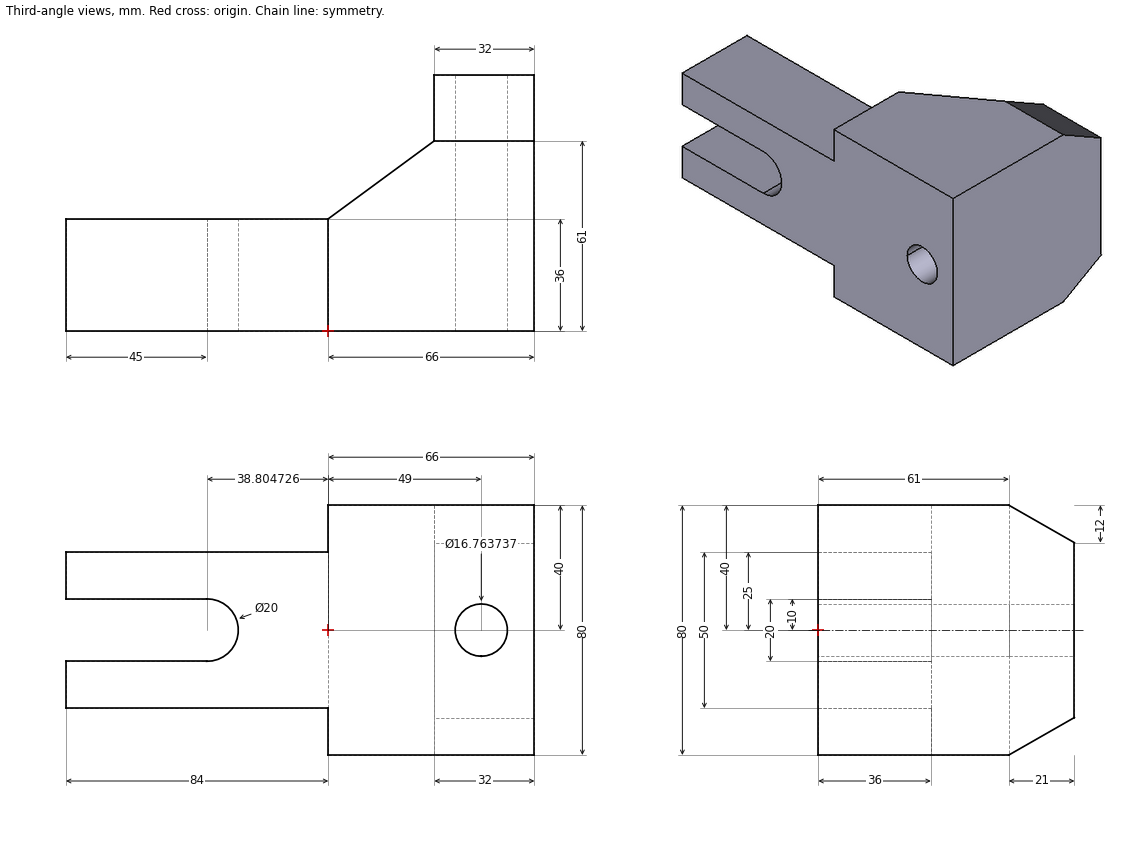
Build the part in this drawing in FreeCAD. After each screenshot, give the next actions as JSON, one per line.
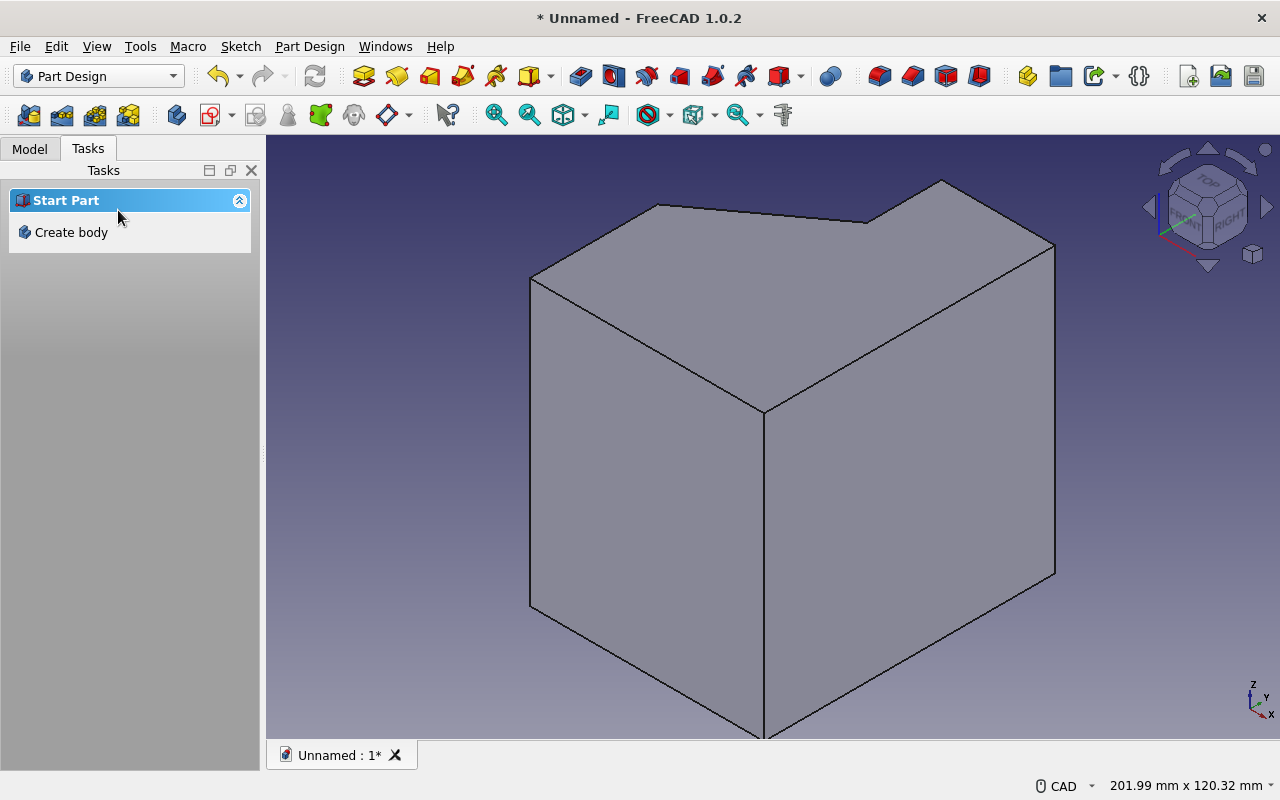
{"action": "left_click", "coordinate": [497, 116]}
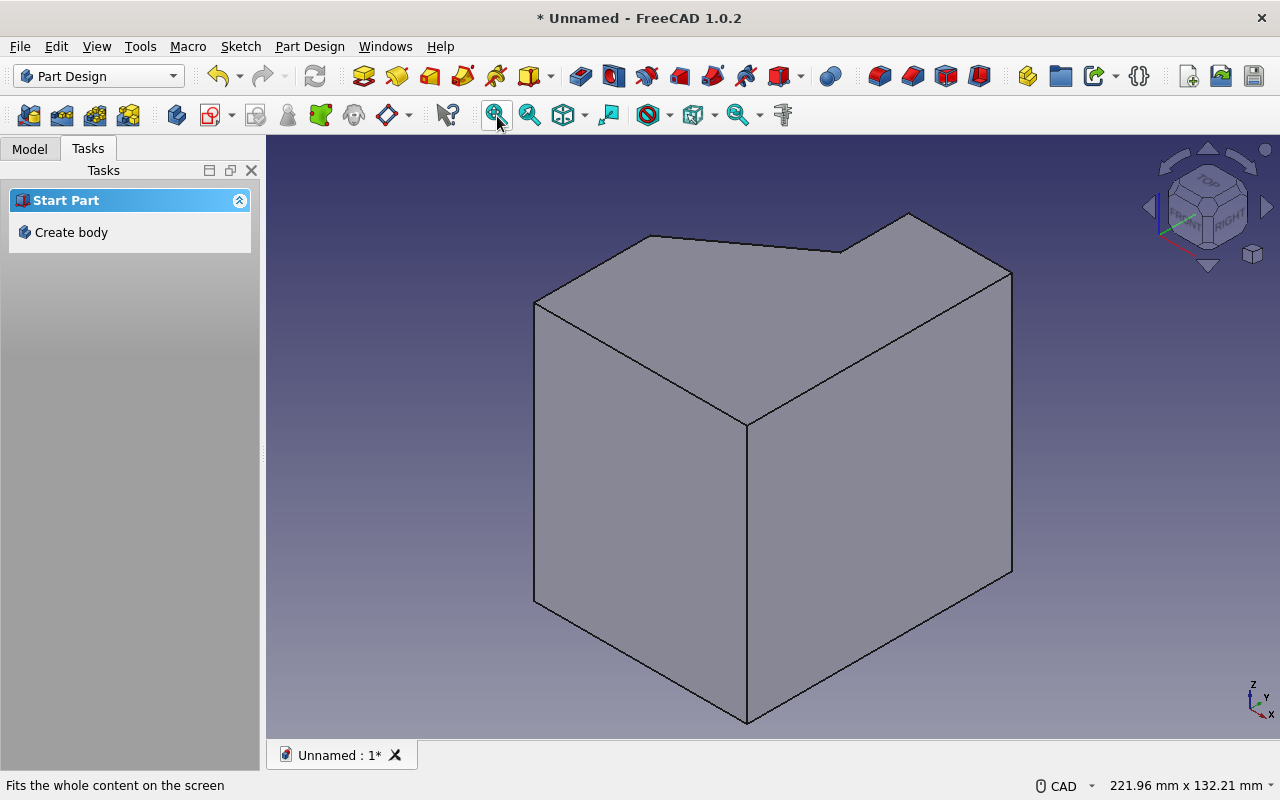
{"action": "left_click", "coordinate": [880, 498]}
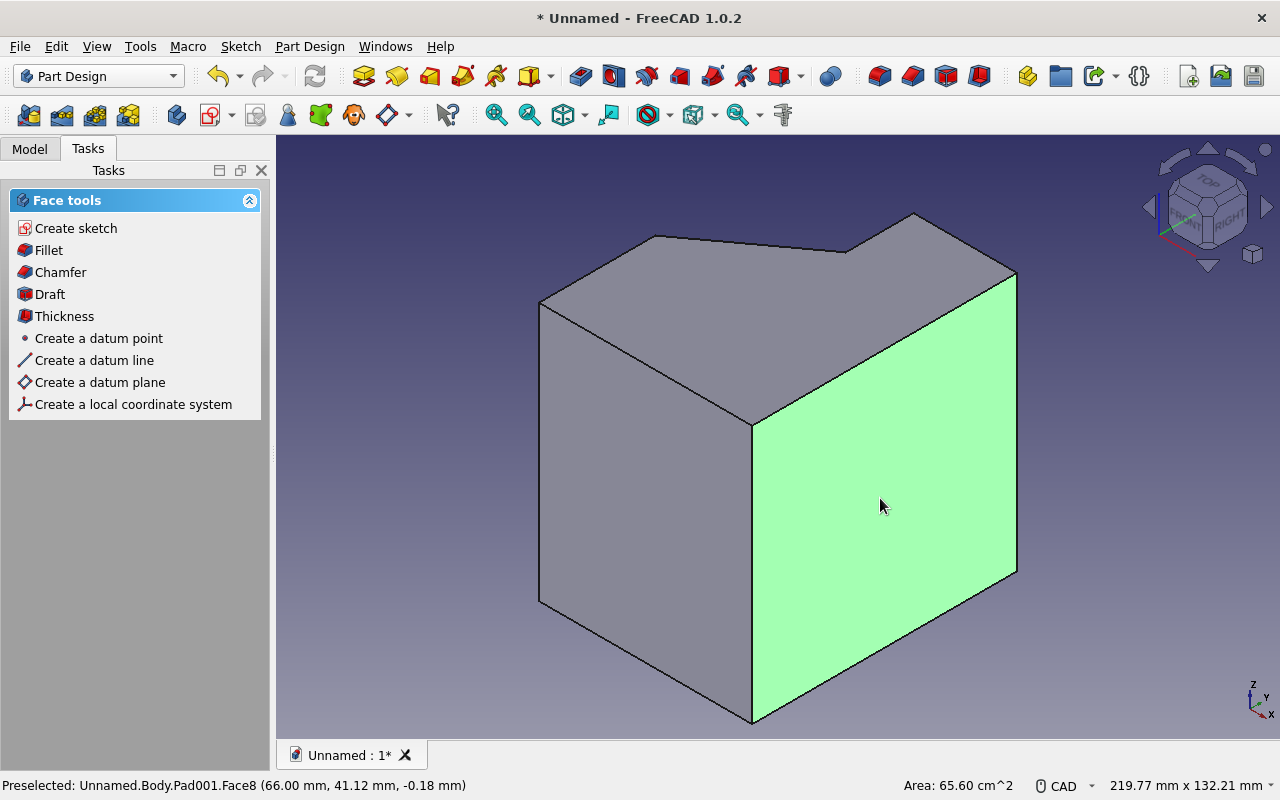
{"action": "left_click", "coordinate": [210, 116]}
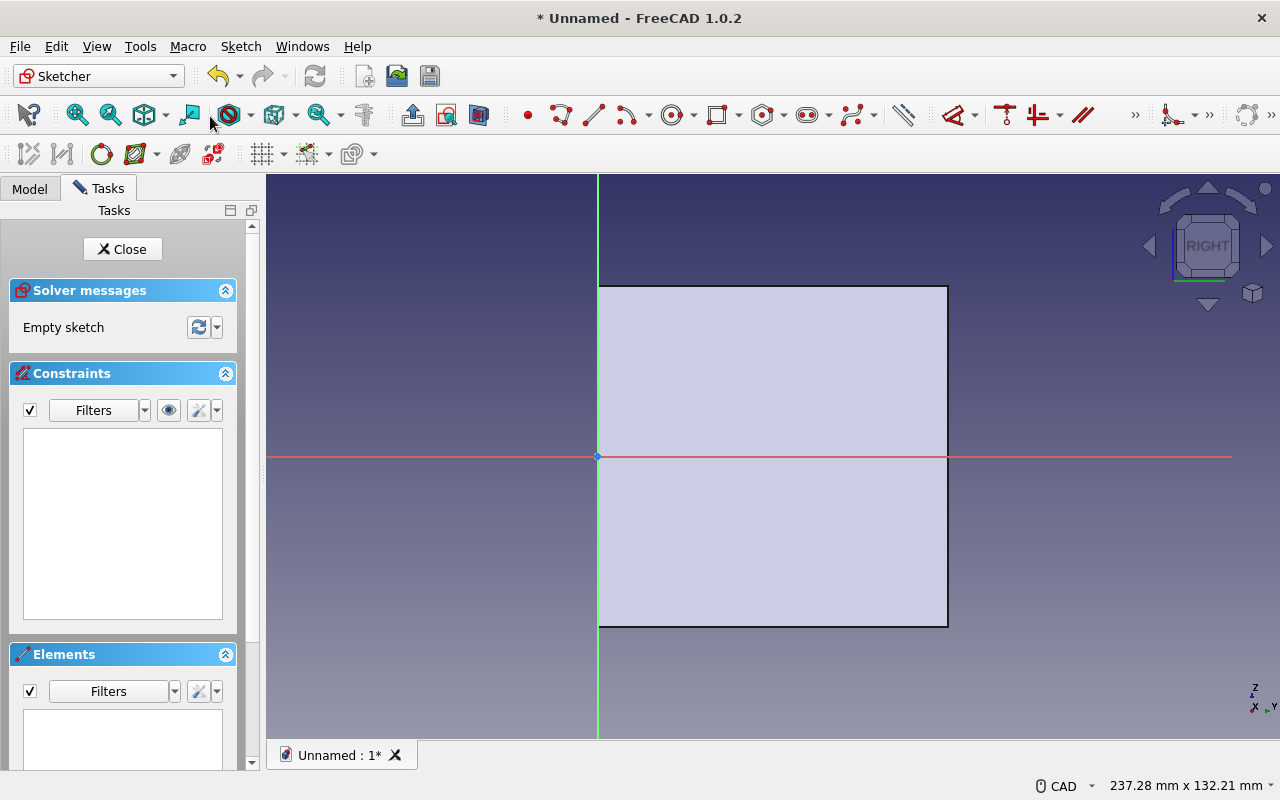
{"action": "key", "text": "g m"}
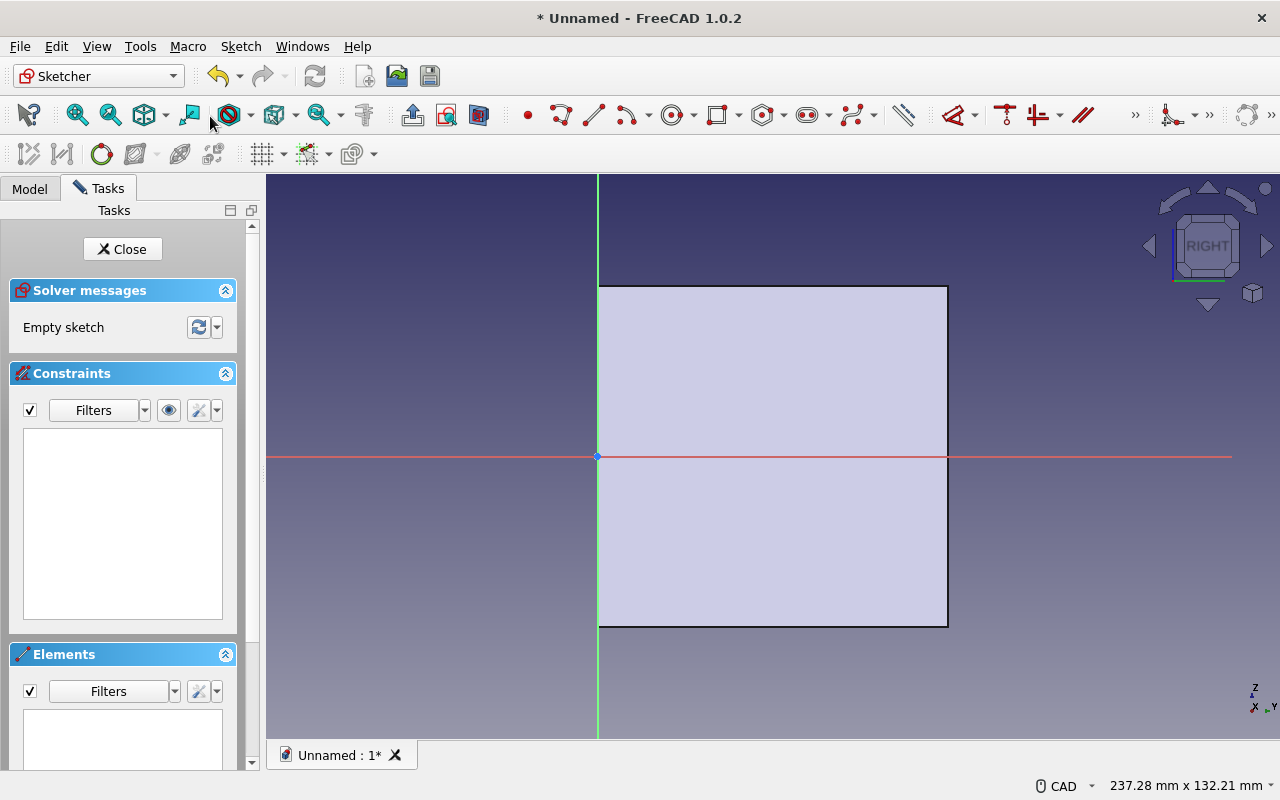
{"action": "left_click", "coordinate": [858, 286]}
{"action": "left_click", "coordinate": [948, 337]}
{"action": "left_click", "coordinate": [948, 286]}
{"action": "left_click", "coordinate": [858, 287]}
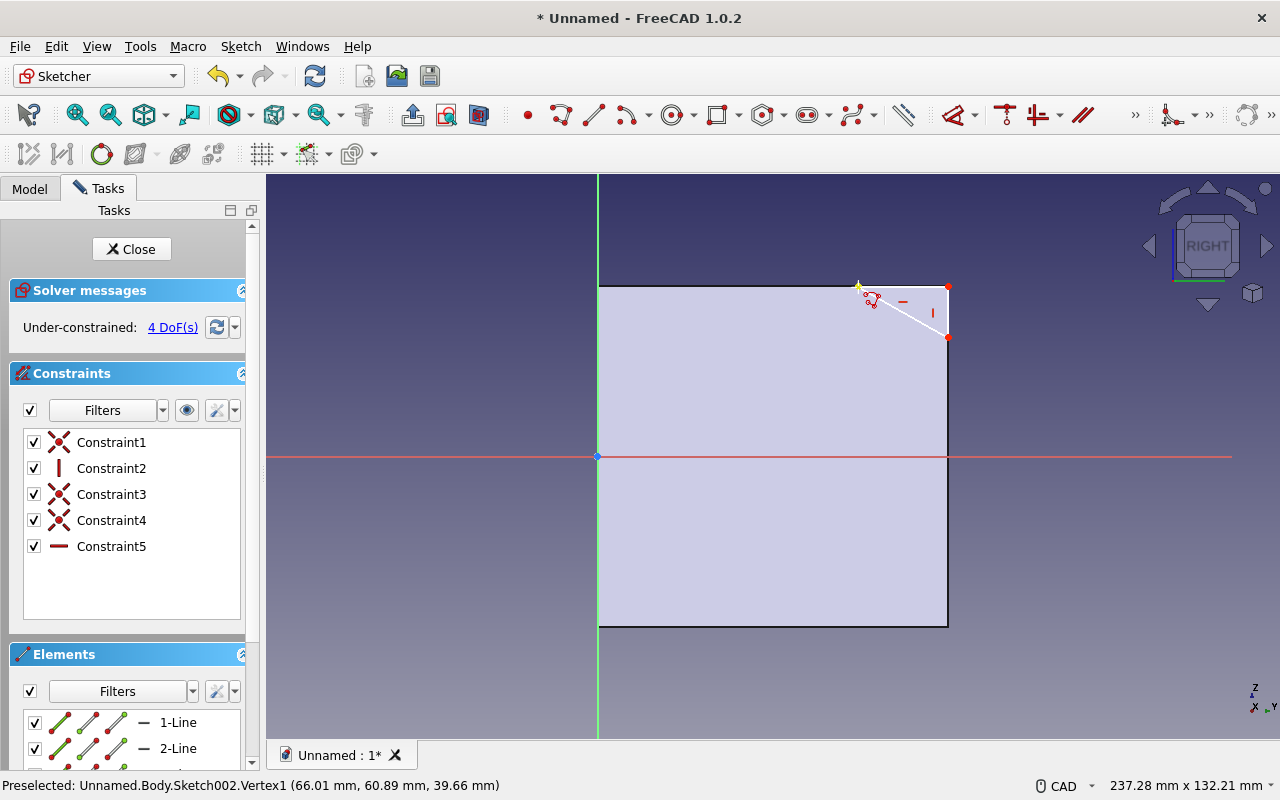
{"action": "left_click", "coordinate": [858, 627]}
{"action": "left_click", "coordinate": [948, 627]}
{"action": "left_click", "coordinate": [948, 576]}
{"action": "left_click", "coordinate": [858, 628]}
{"action": "key", "text": "Escape"}
{"action": "key", "text": "Escape"}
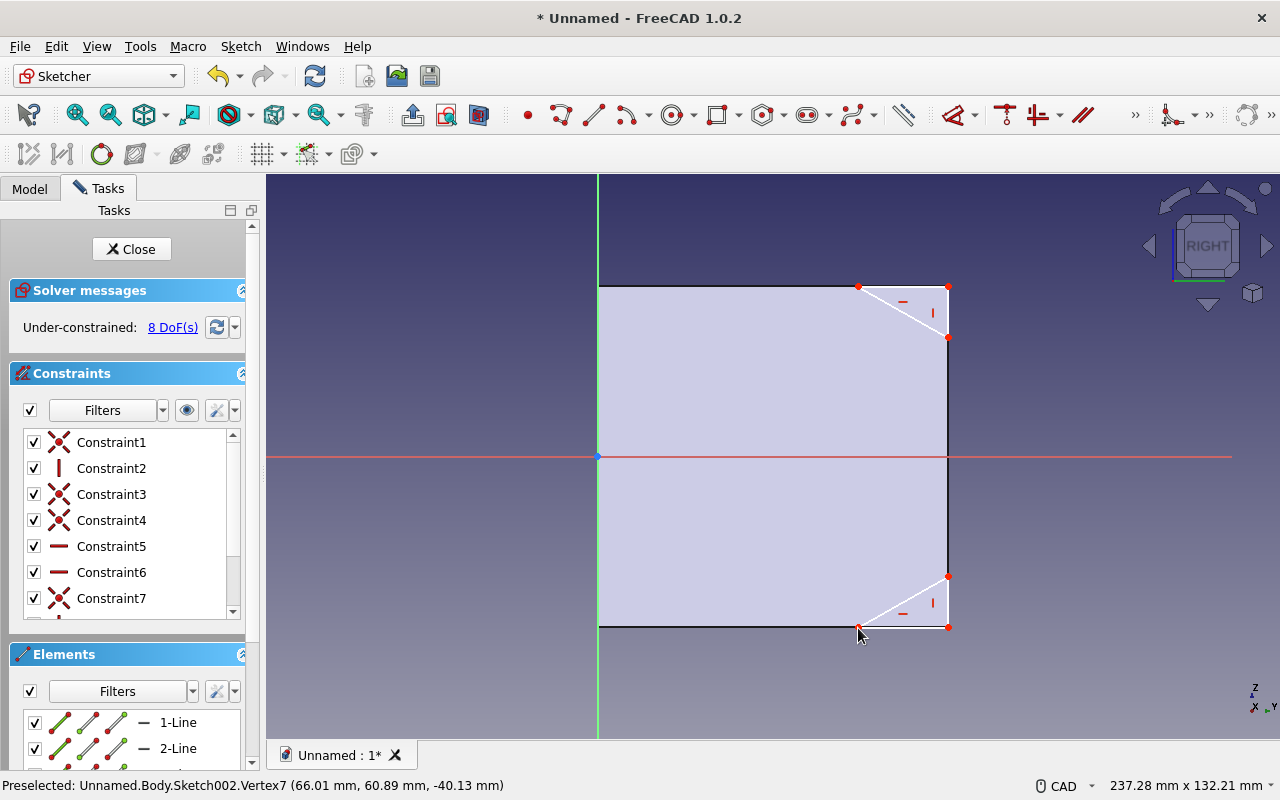
{"action": "left_click", "coordinate": [858, 287]}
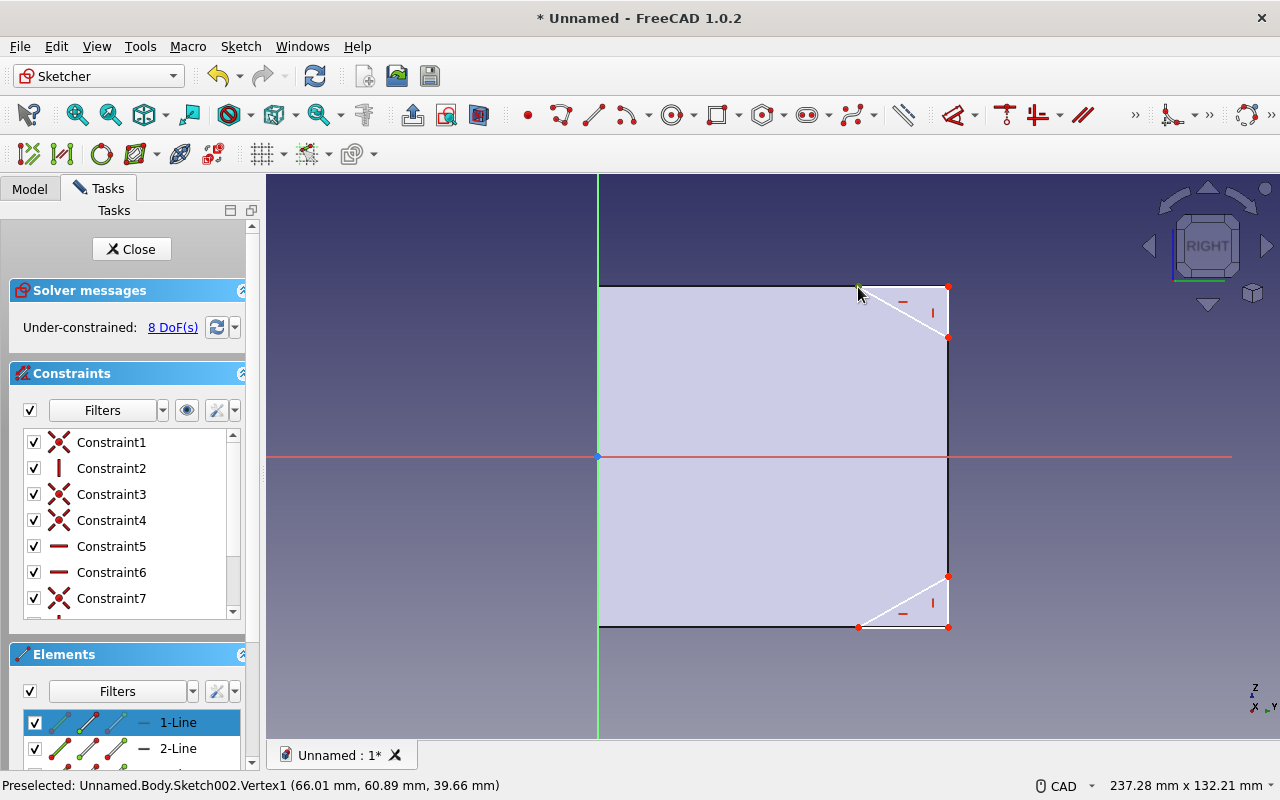
{"action": "left_click", "coordinate": [858, 628]}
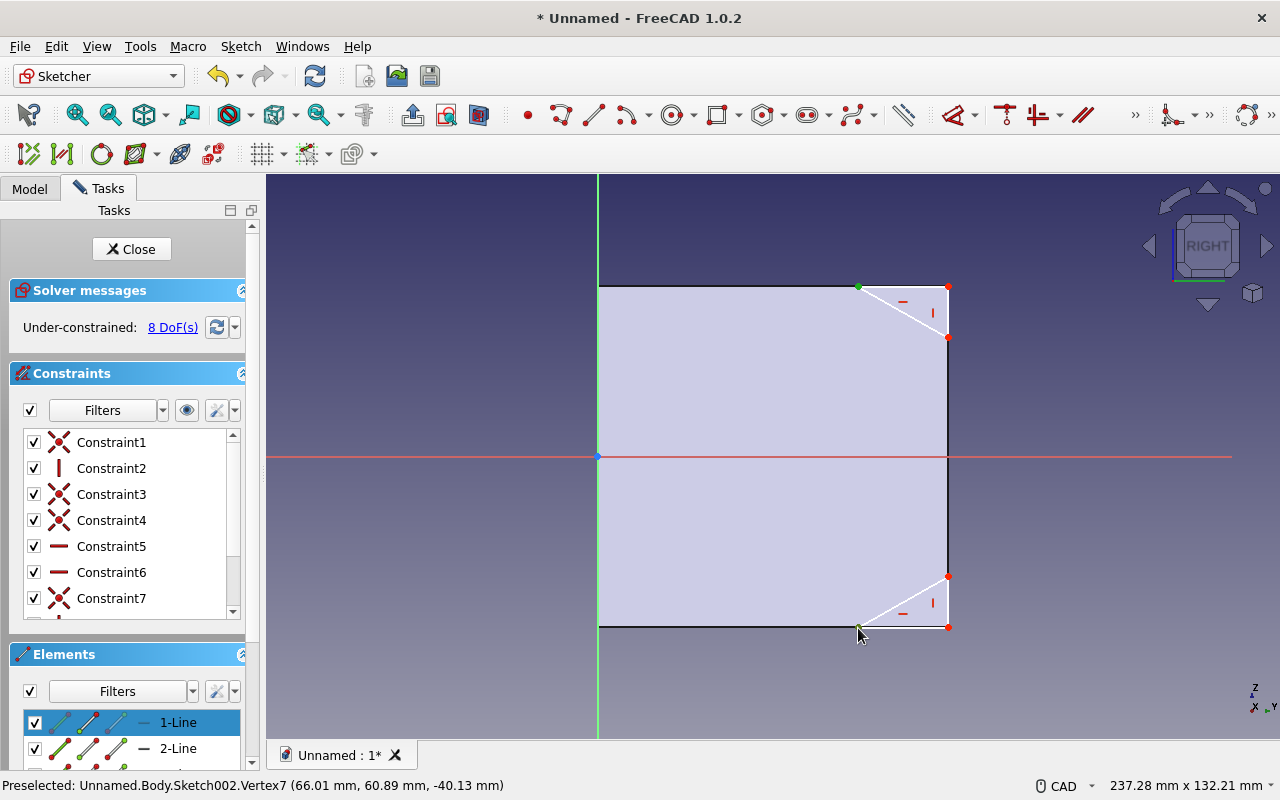
{"action": "left_click", "coordinate": [353, 456]}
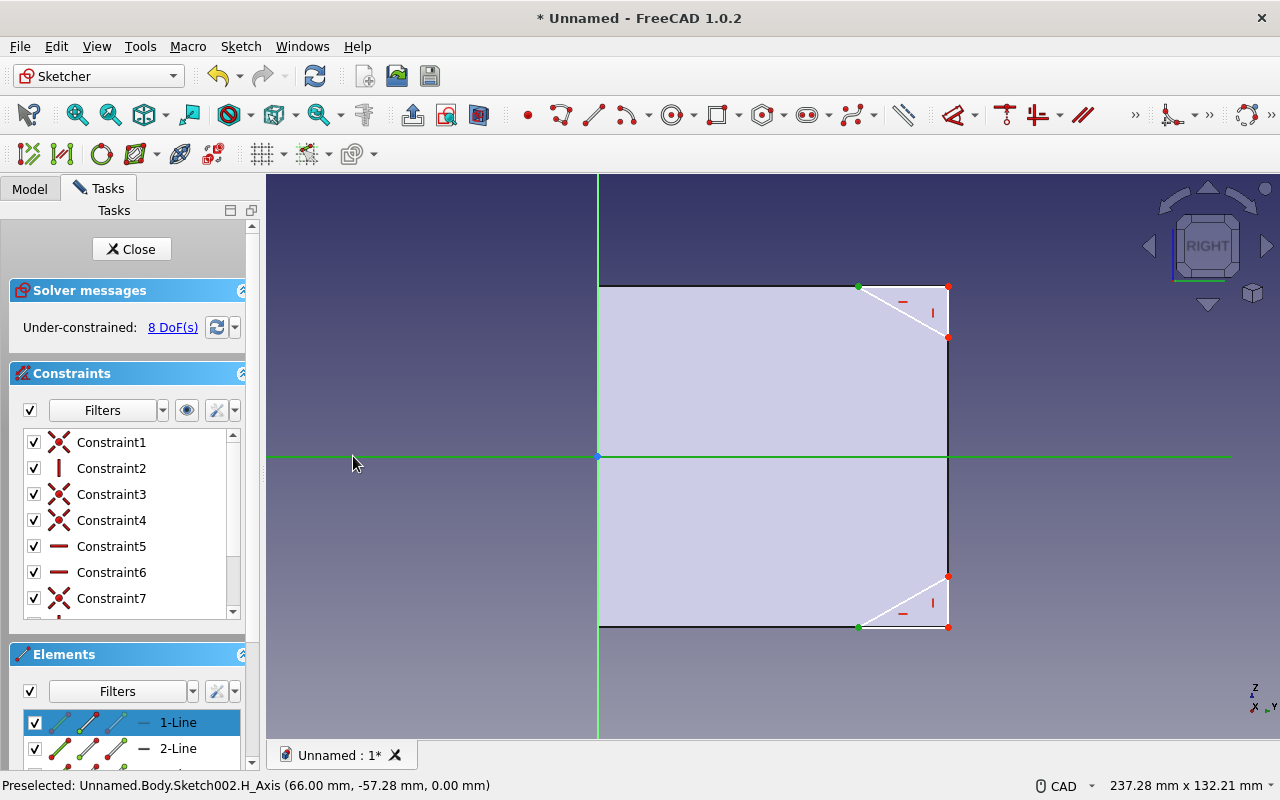
{"action": "key", "text": "s"}